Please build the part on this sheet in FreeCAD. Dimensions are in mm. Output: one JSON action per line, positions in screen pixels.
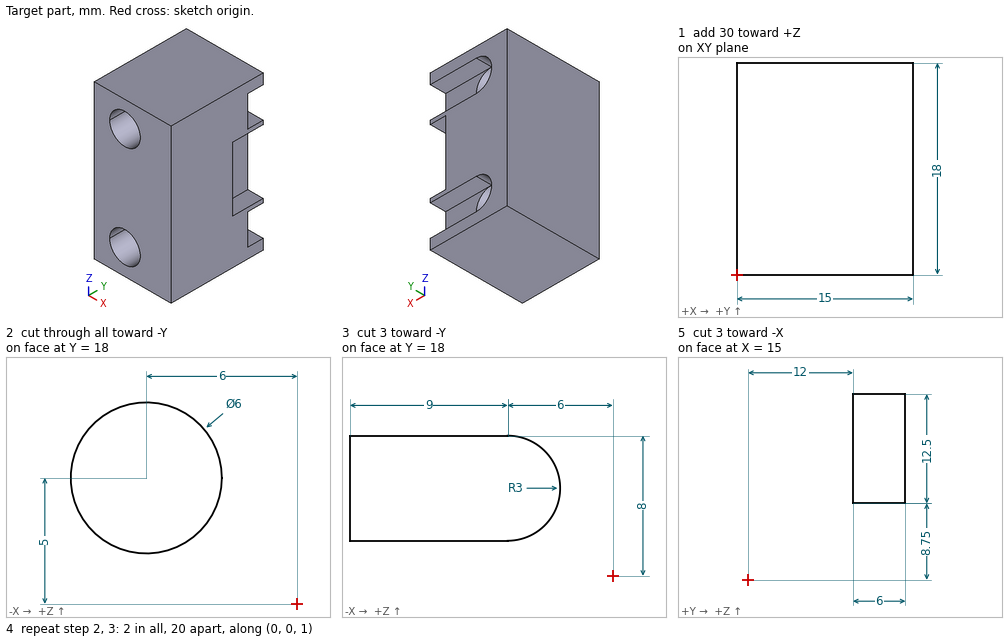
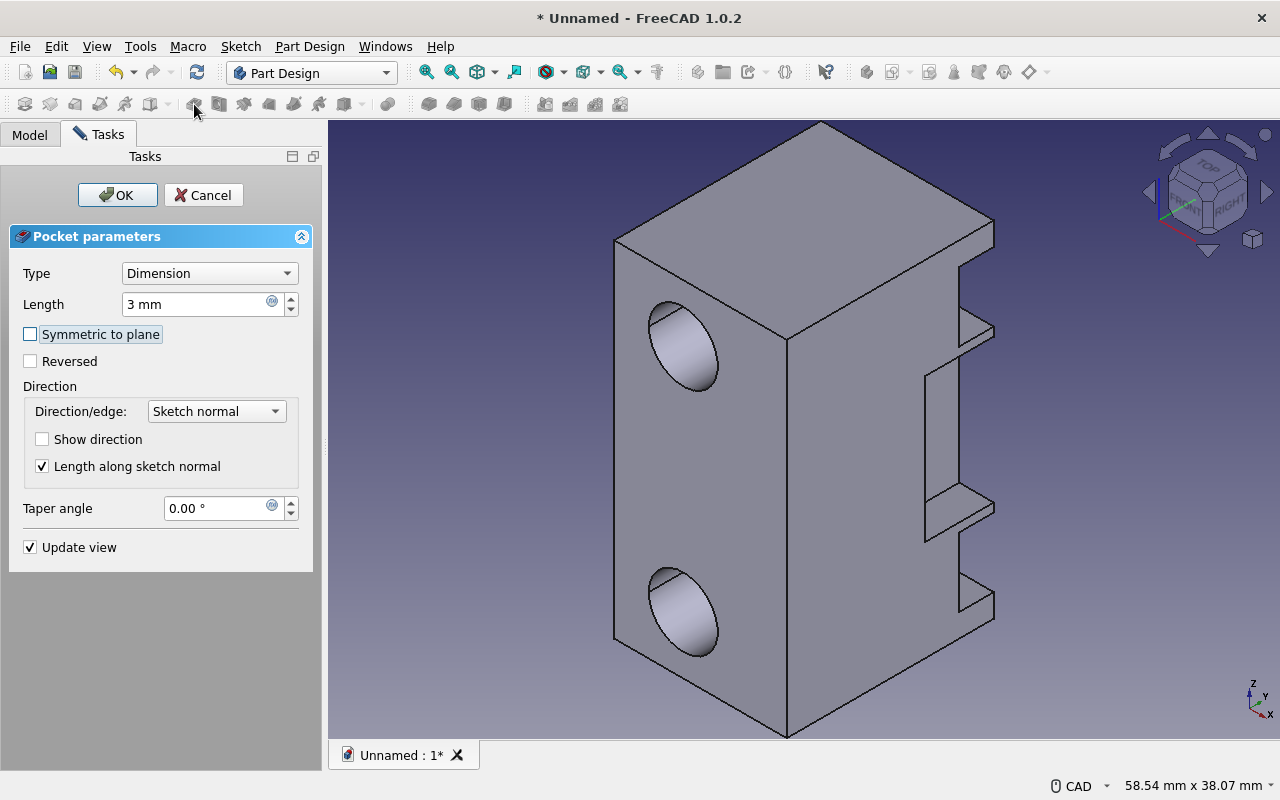
{"action": "left_click", "coordinate": [118, 195]}